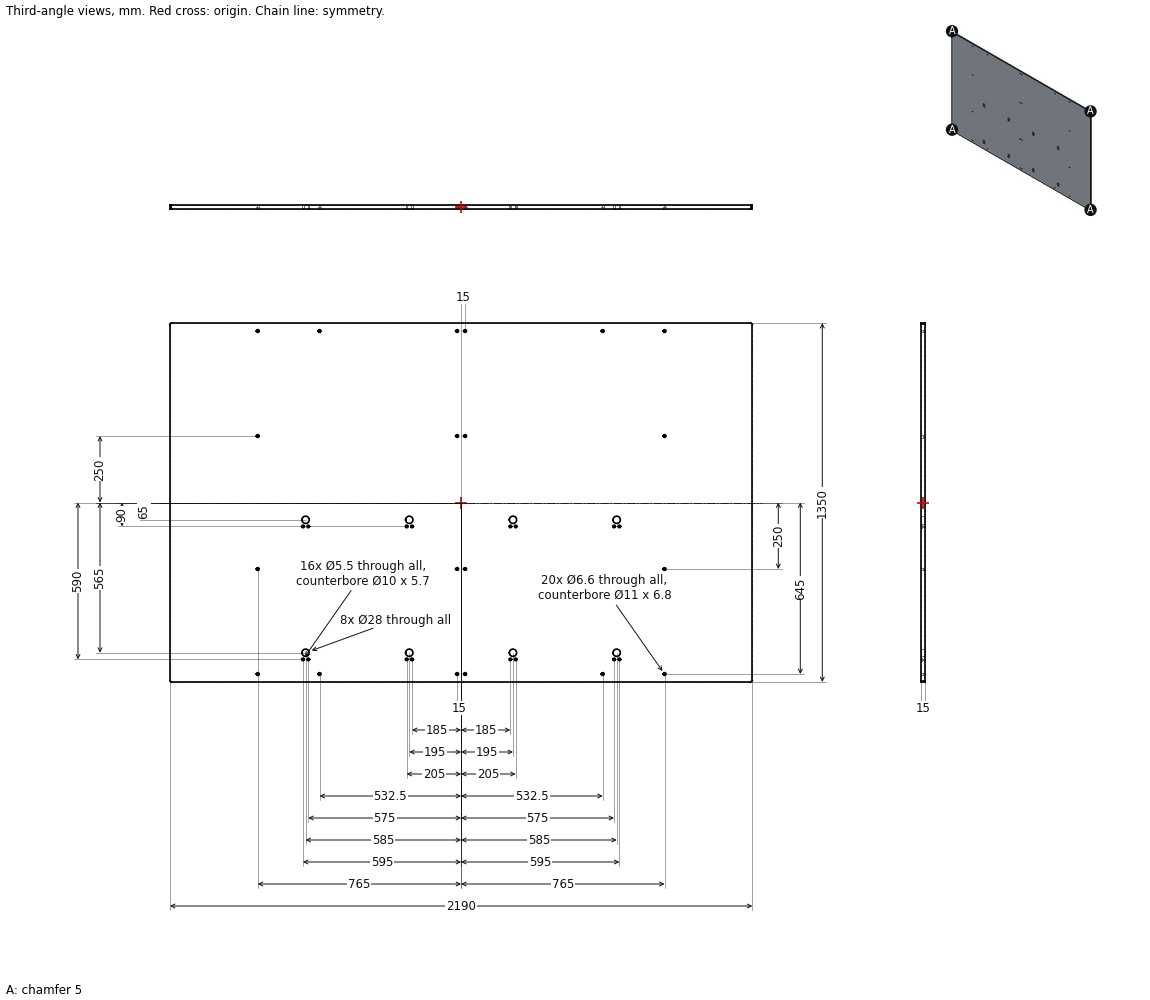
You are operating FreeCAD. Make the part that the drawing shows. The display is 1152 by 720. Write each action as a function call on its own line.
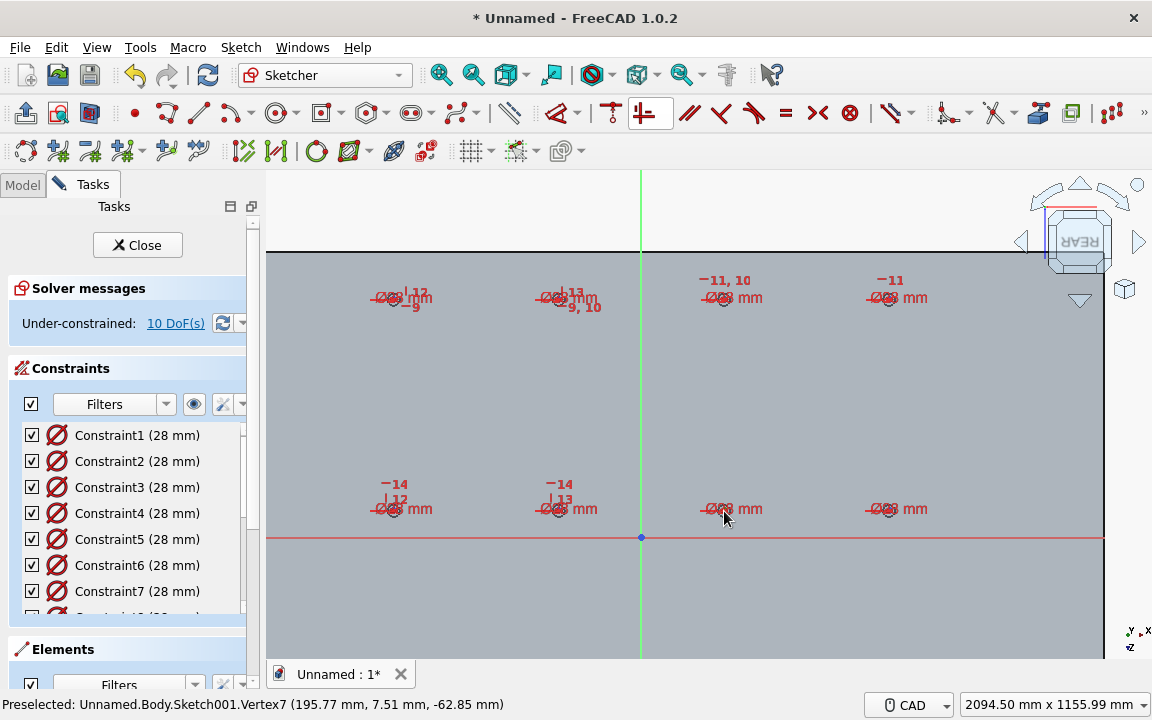
click(668, 114)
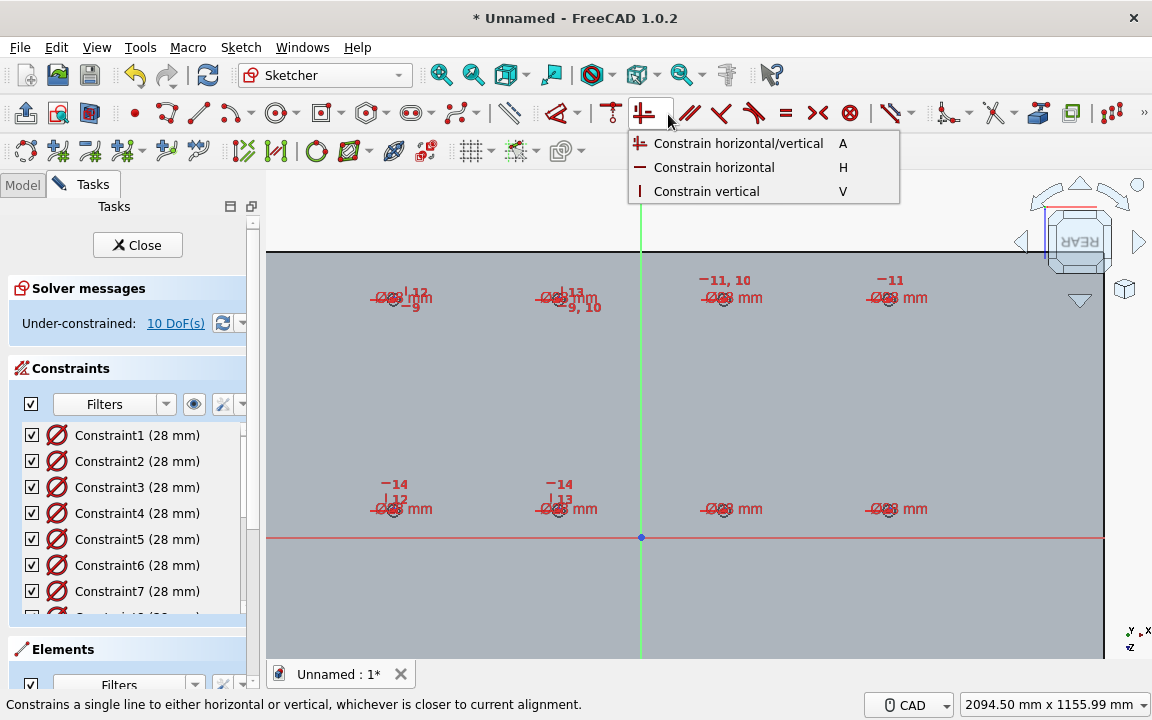
click(764, 191)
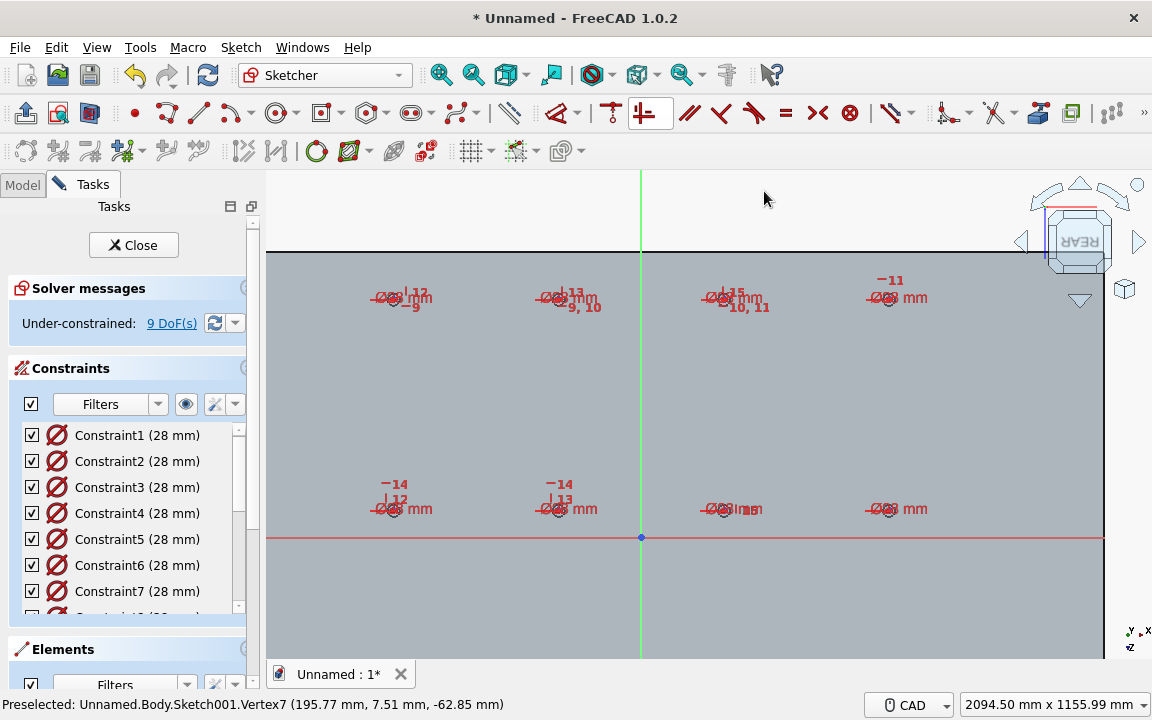
click(559, 511)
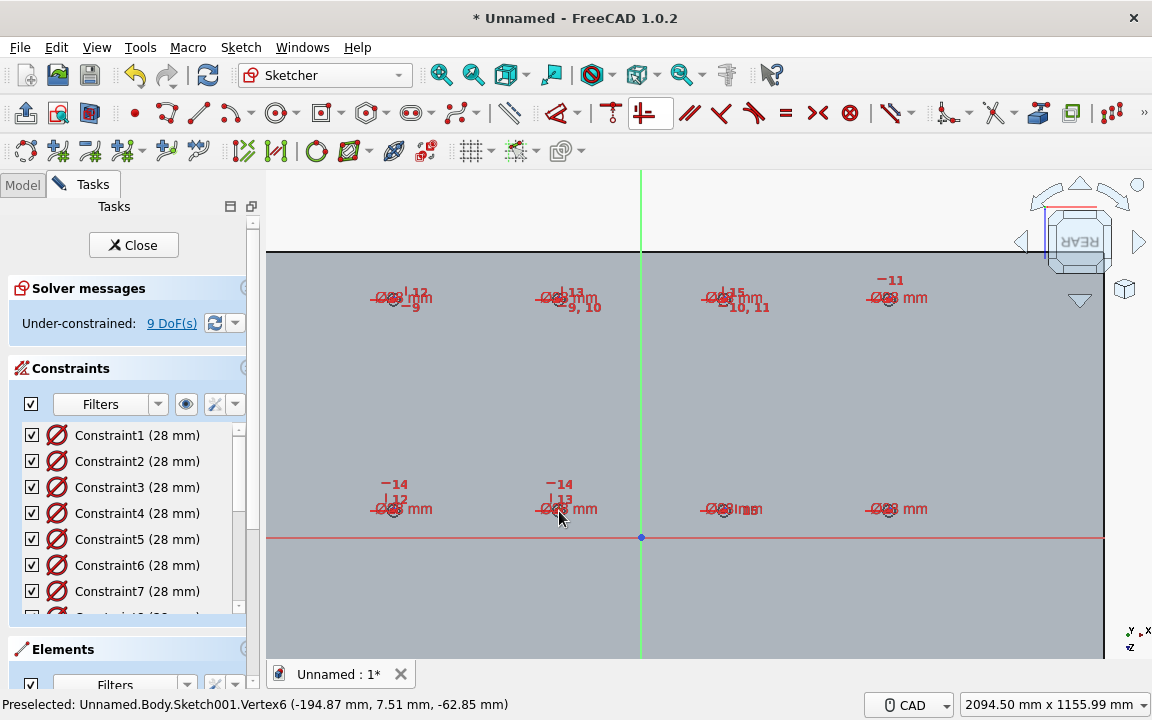
click(724, 511)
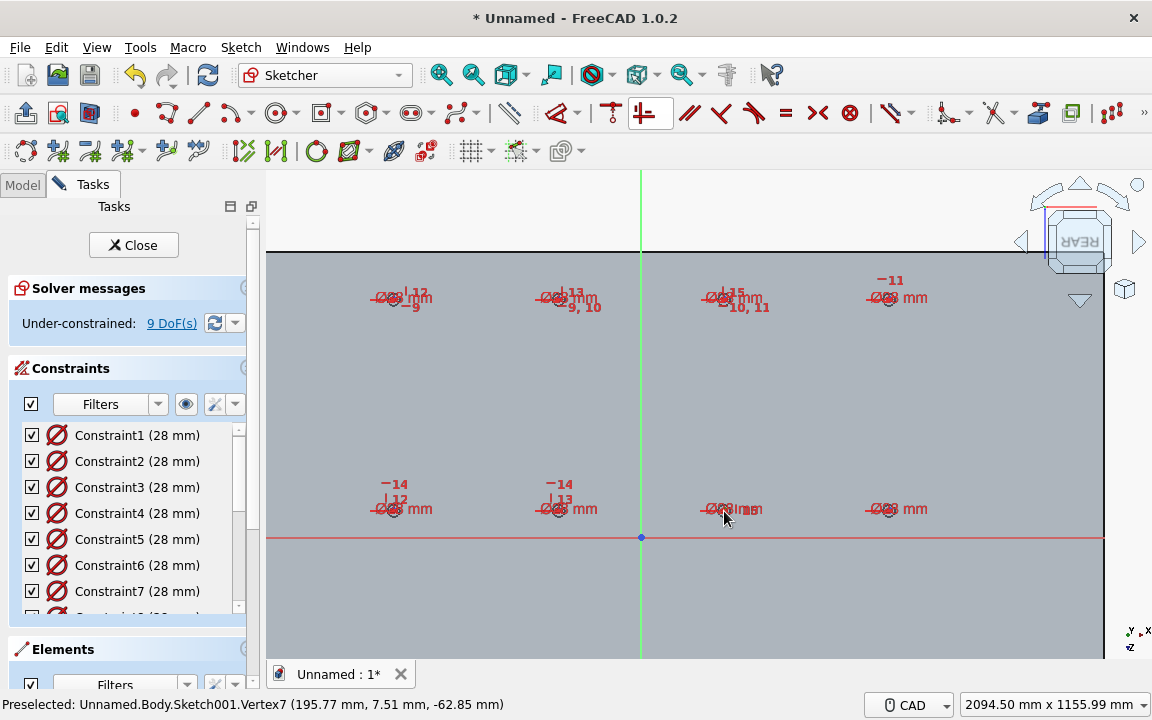
key(h)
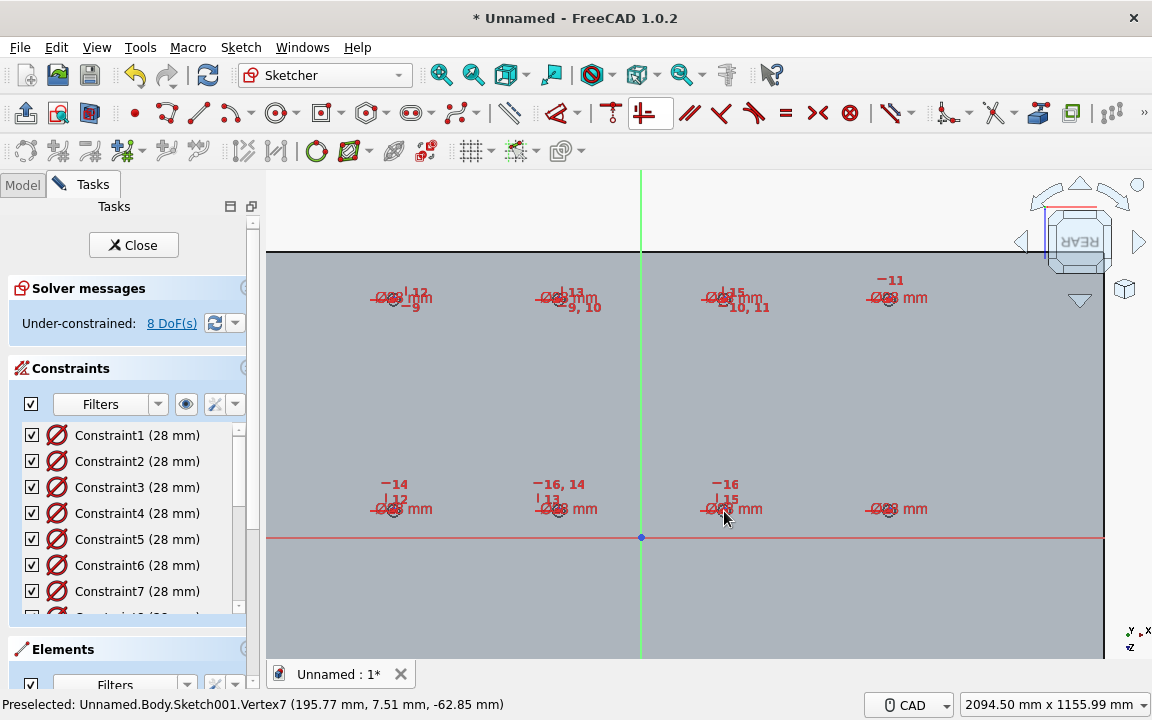
click(889, 300)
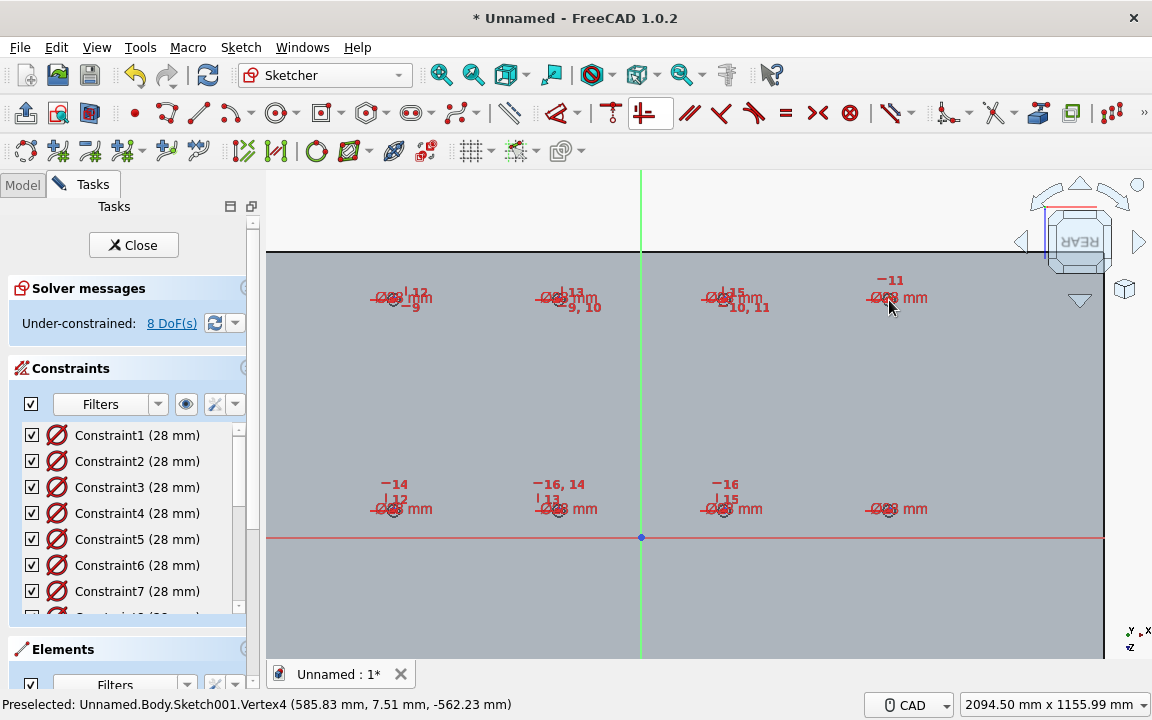
click(889, 511)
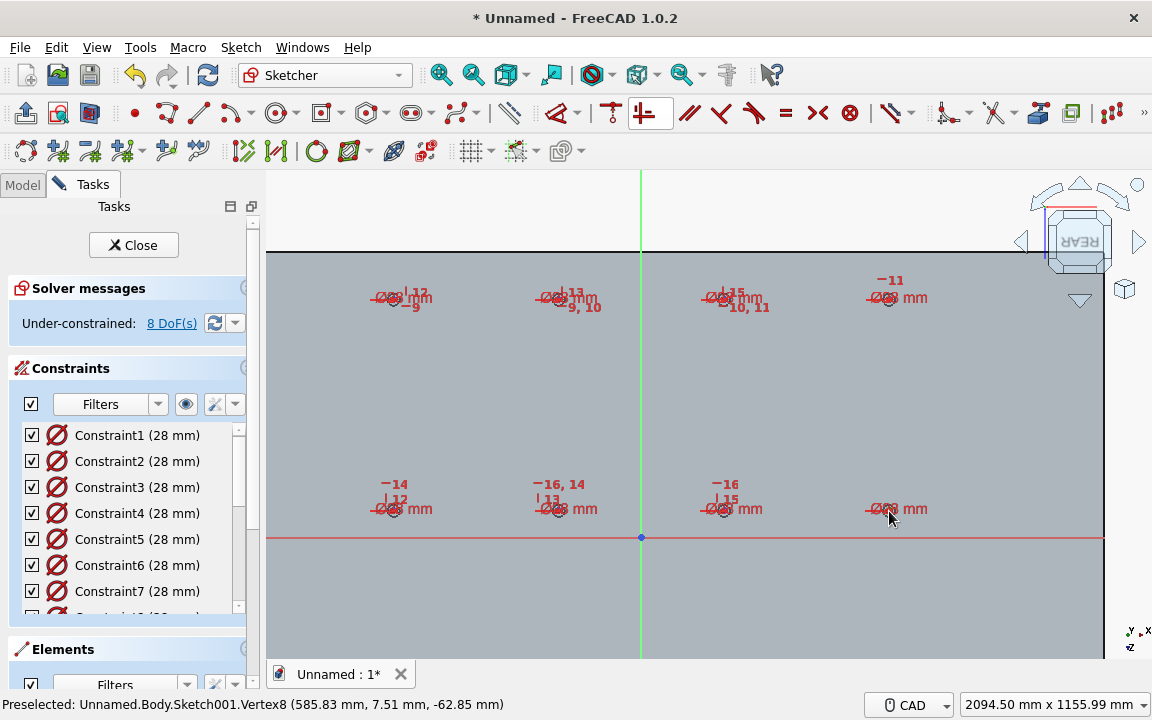
click(668, 114)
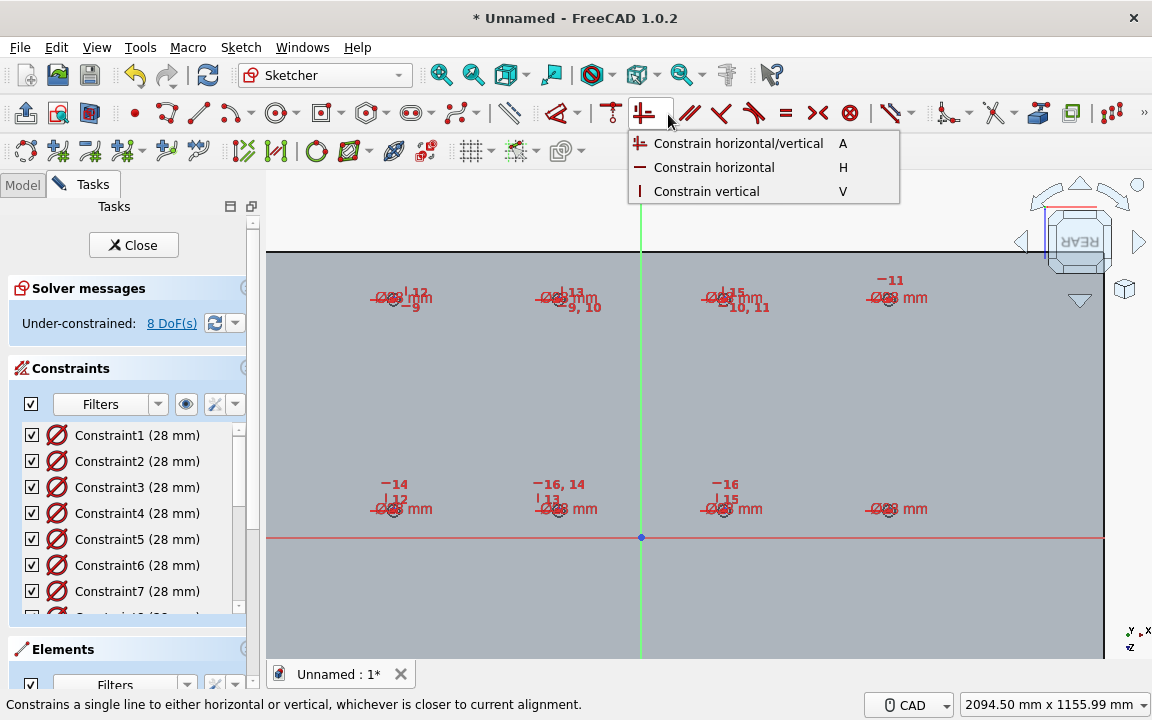
click(764, 191)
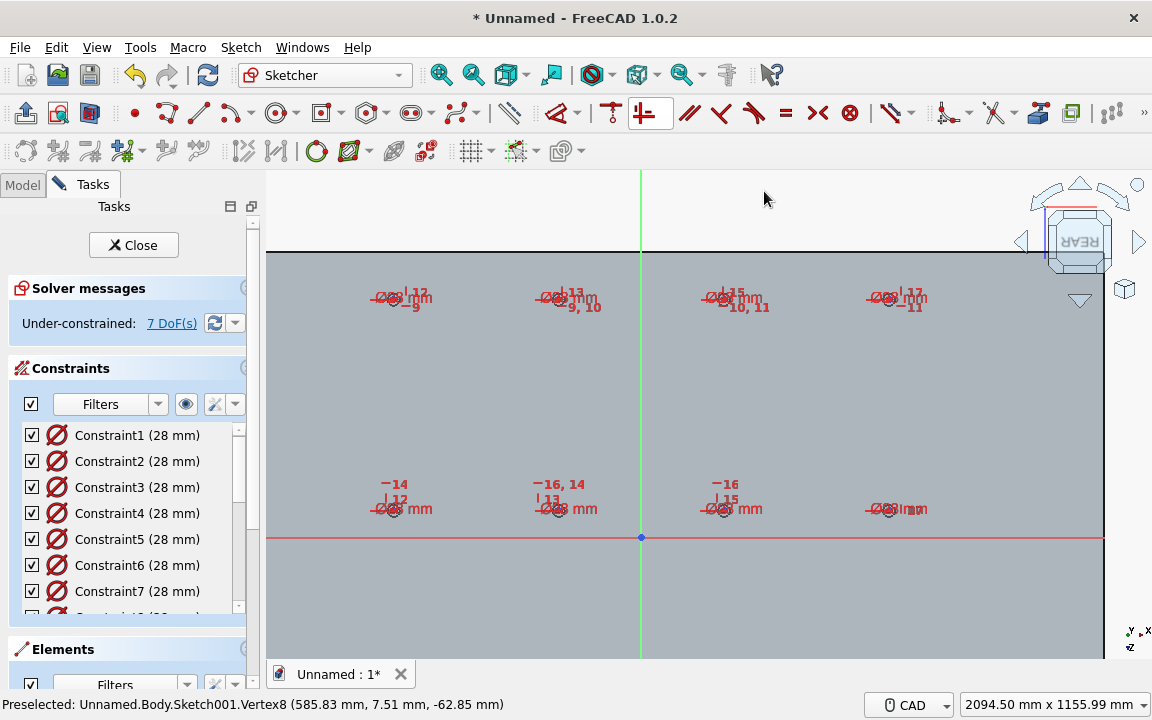
click(724, 511)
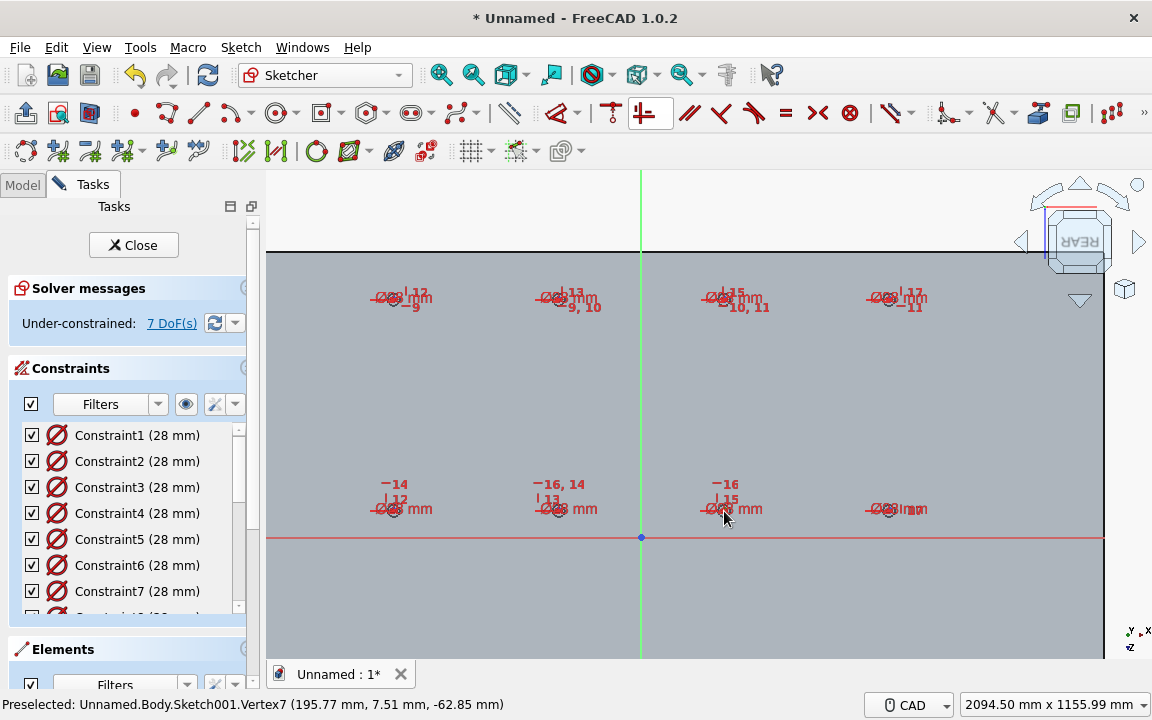
click(889, 511)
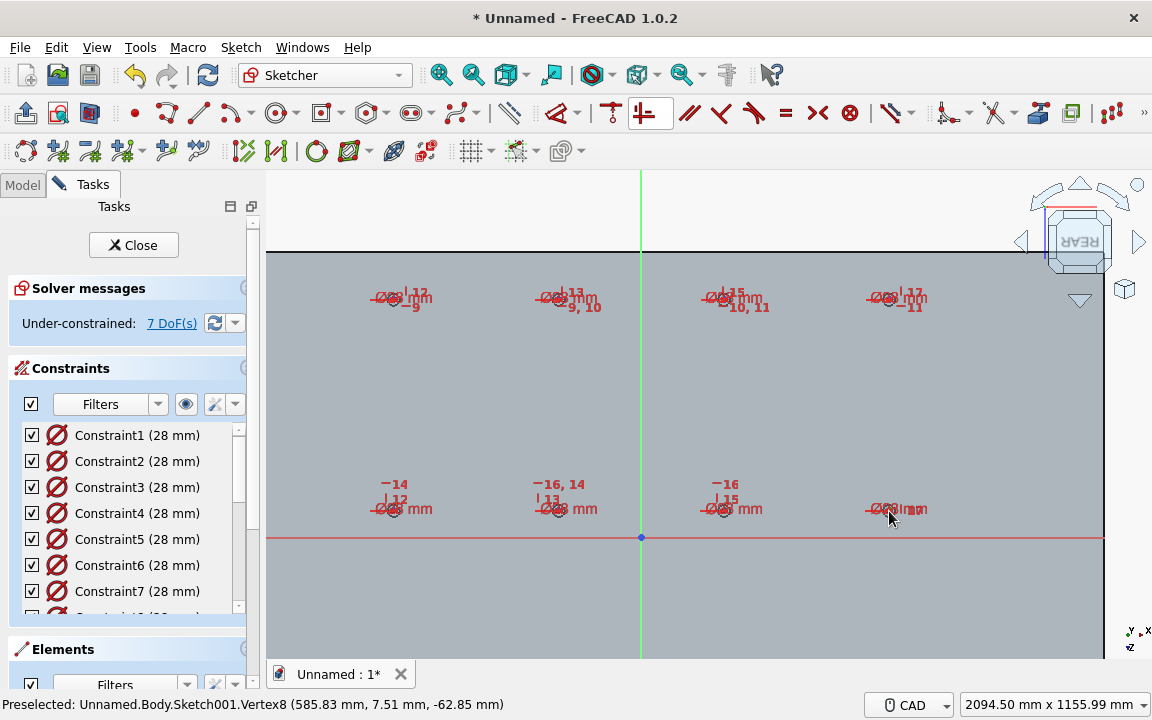
key(h)